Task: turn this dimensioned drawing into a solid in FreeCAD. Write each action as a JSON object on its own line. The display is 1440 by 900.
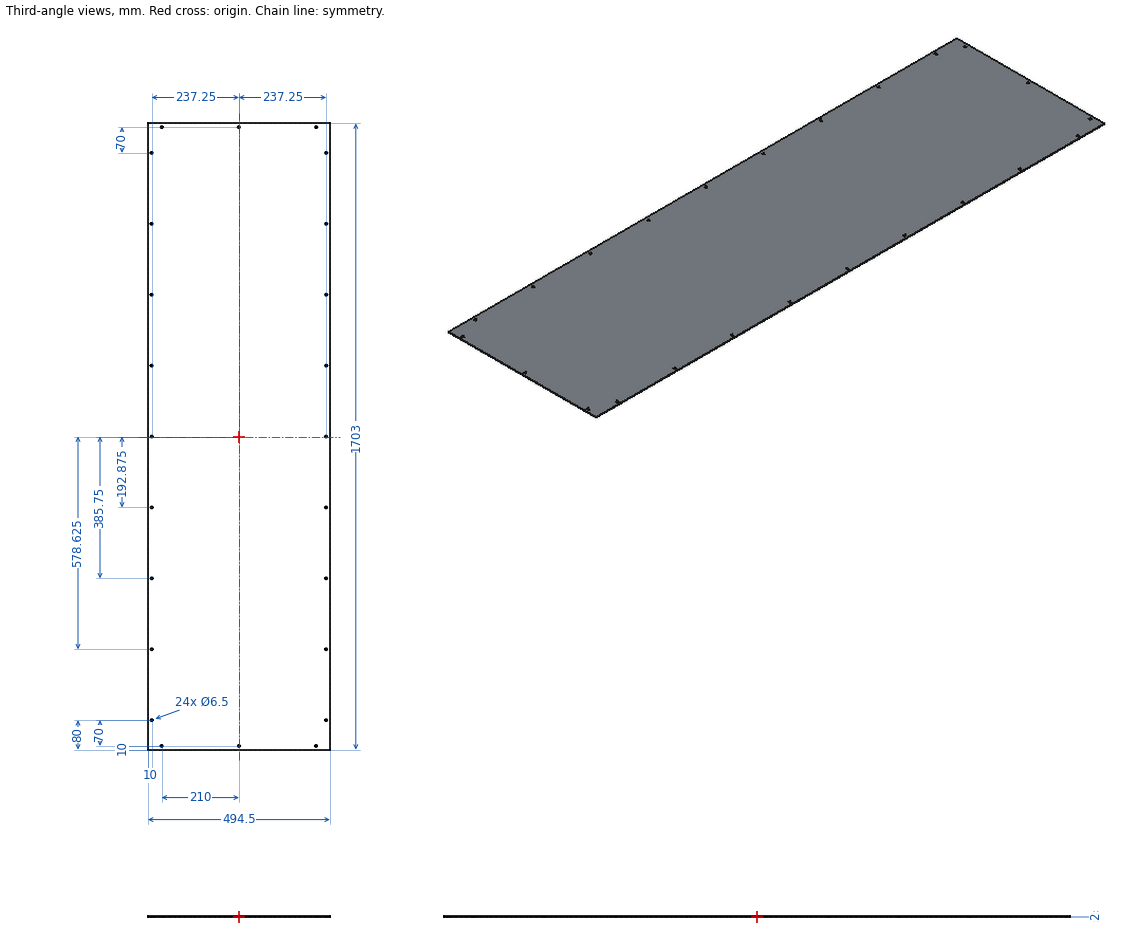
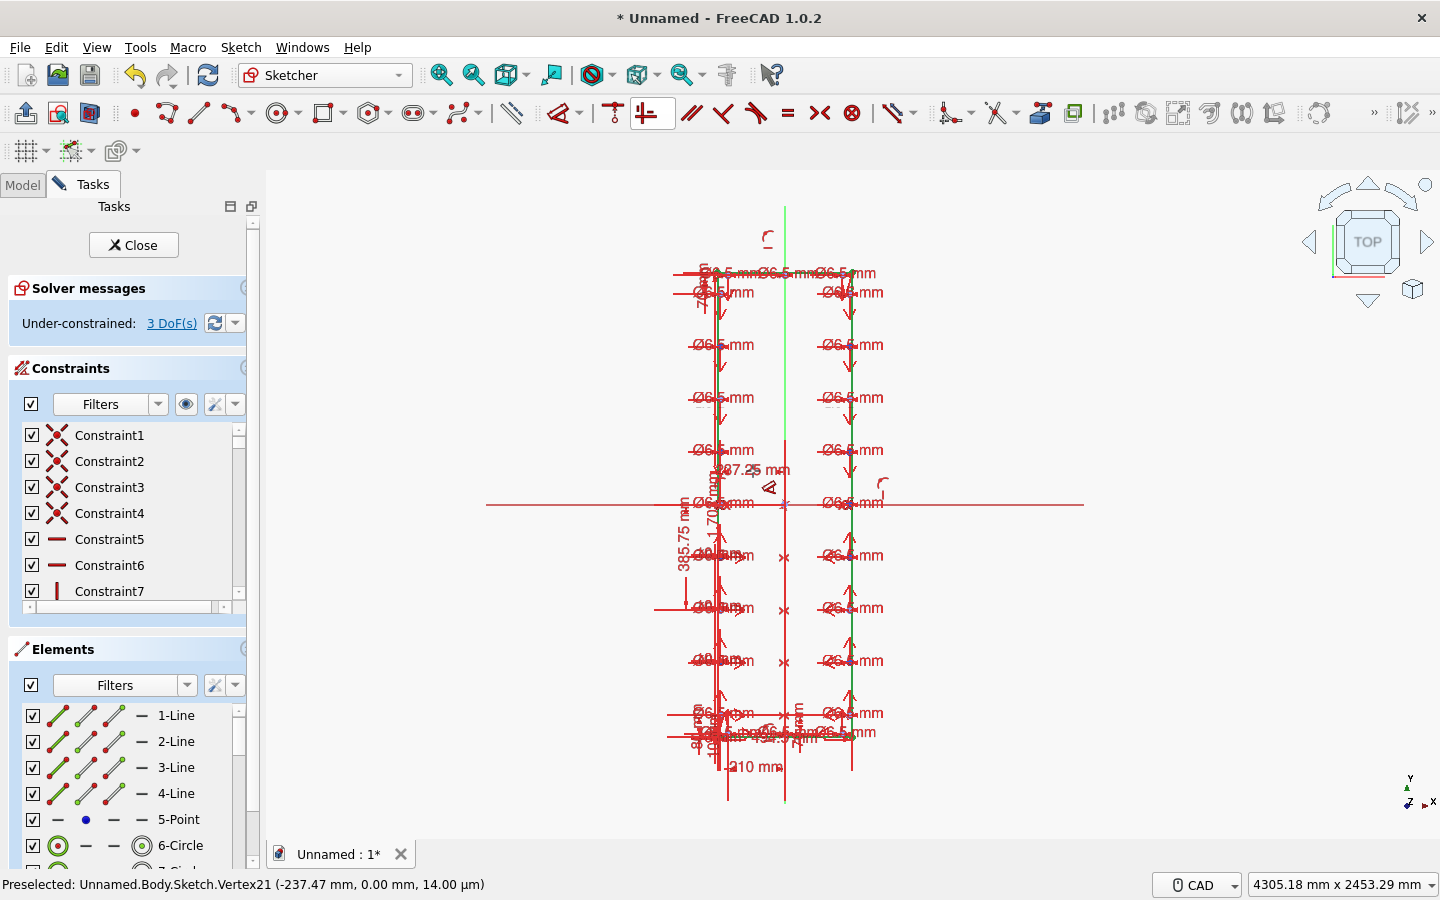
{"action": "left_click", "coordinate": [850, 505]}
{"action": "left_click", "coordinate": [817, 539]}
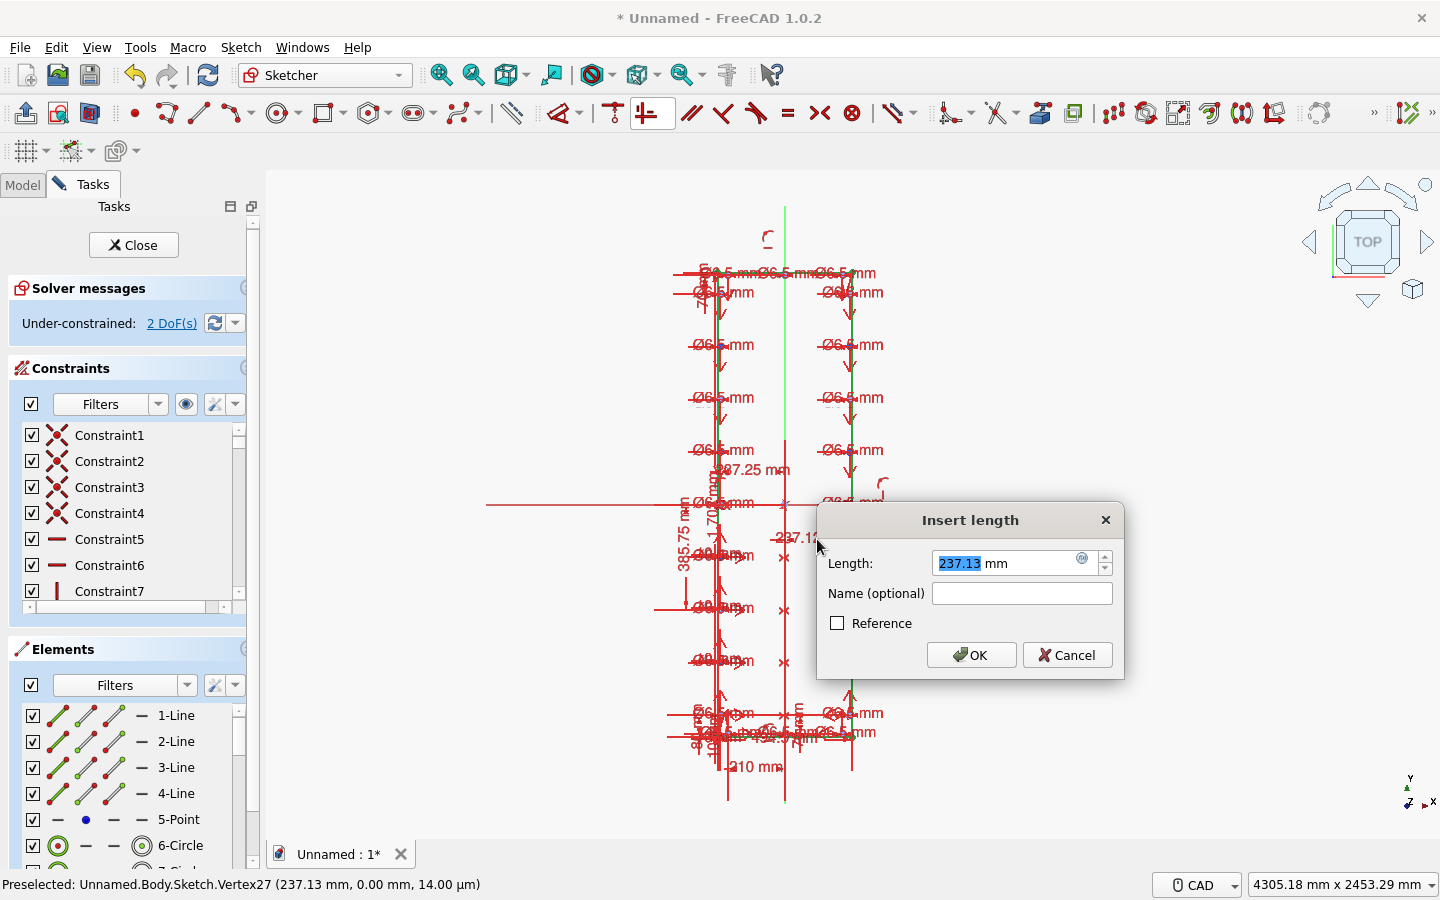
{"action": "type", "text": "237.25"}
{"action": "key", "text": "Return"}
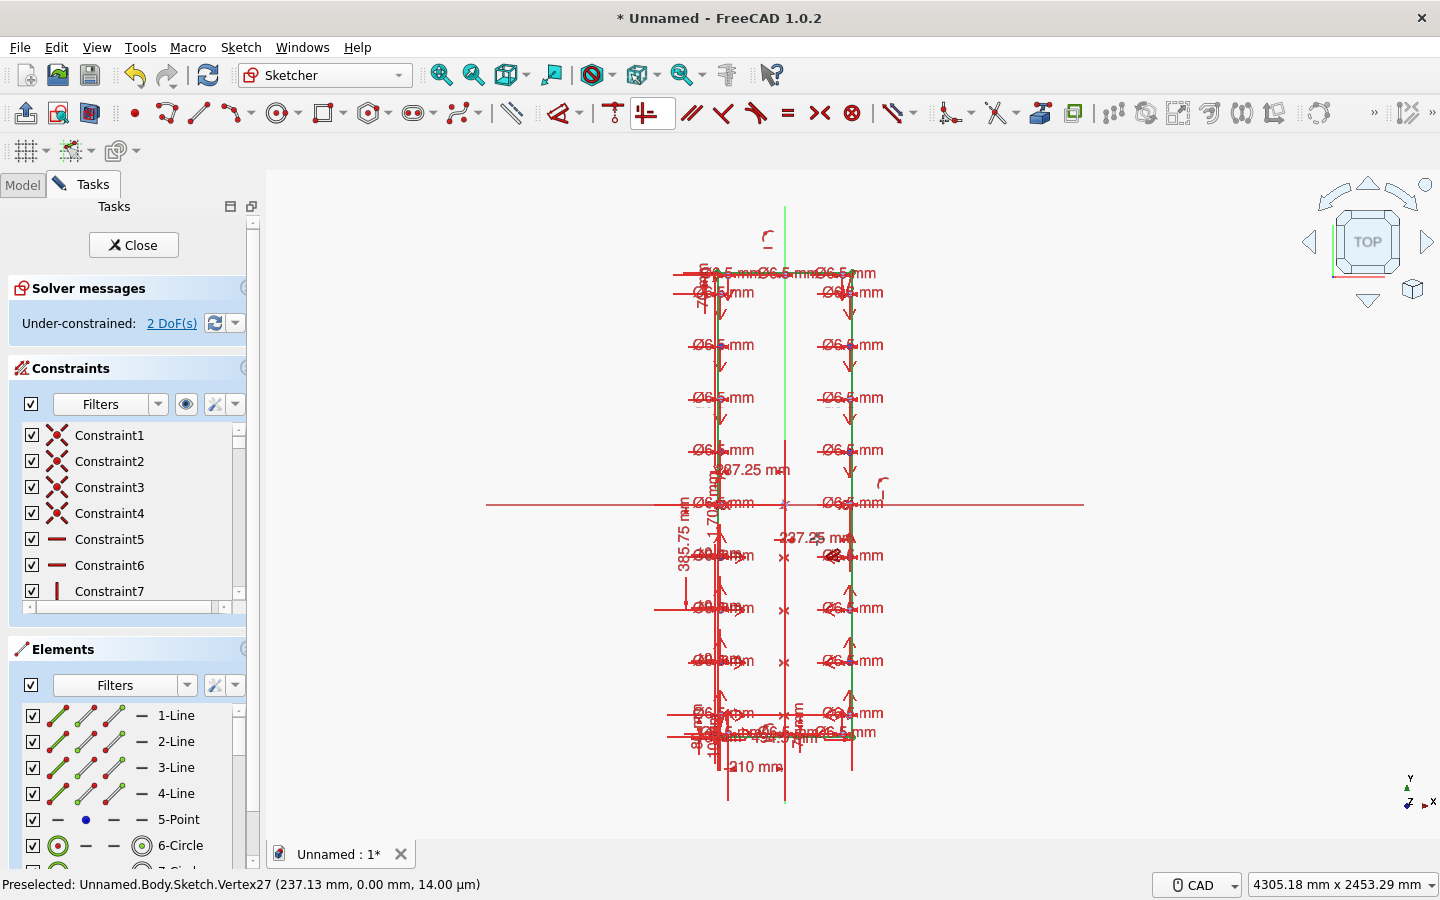
{"action": "left_click", "coordinate": [720, 663]}
{"action": "left_click", "coordinate": [686, 584]}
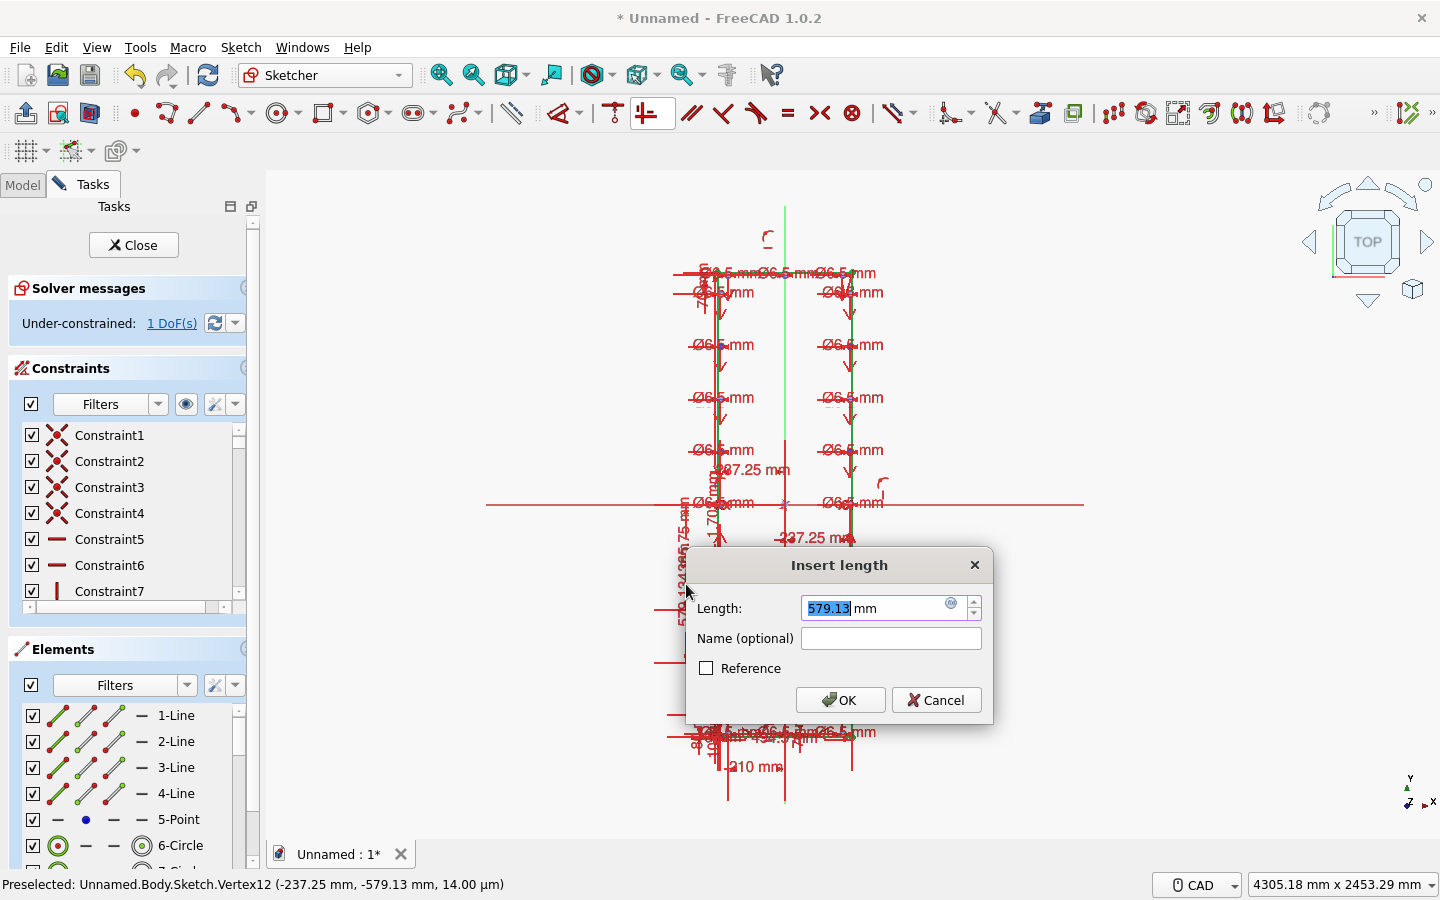
{"action": "type", "text": "578.625"}
{"action": "key", "text": "Return"}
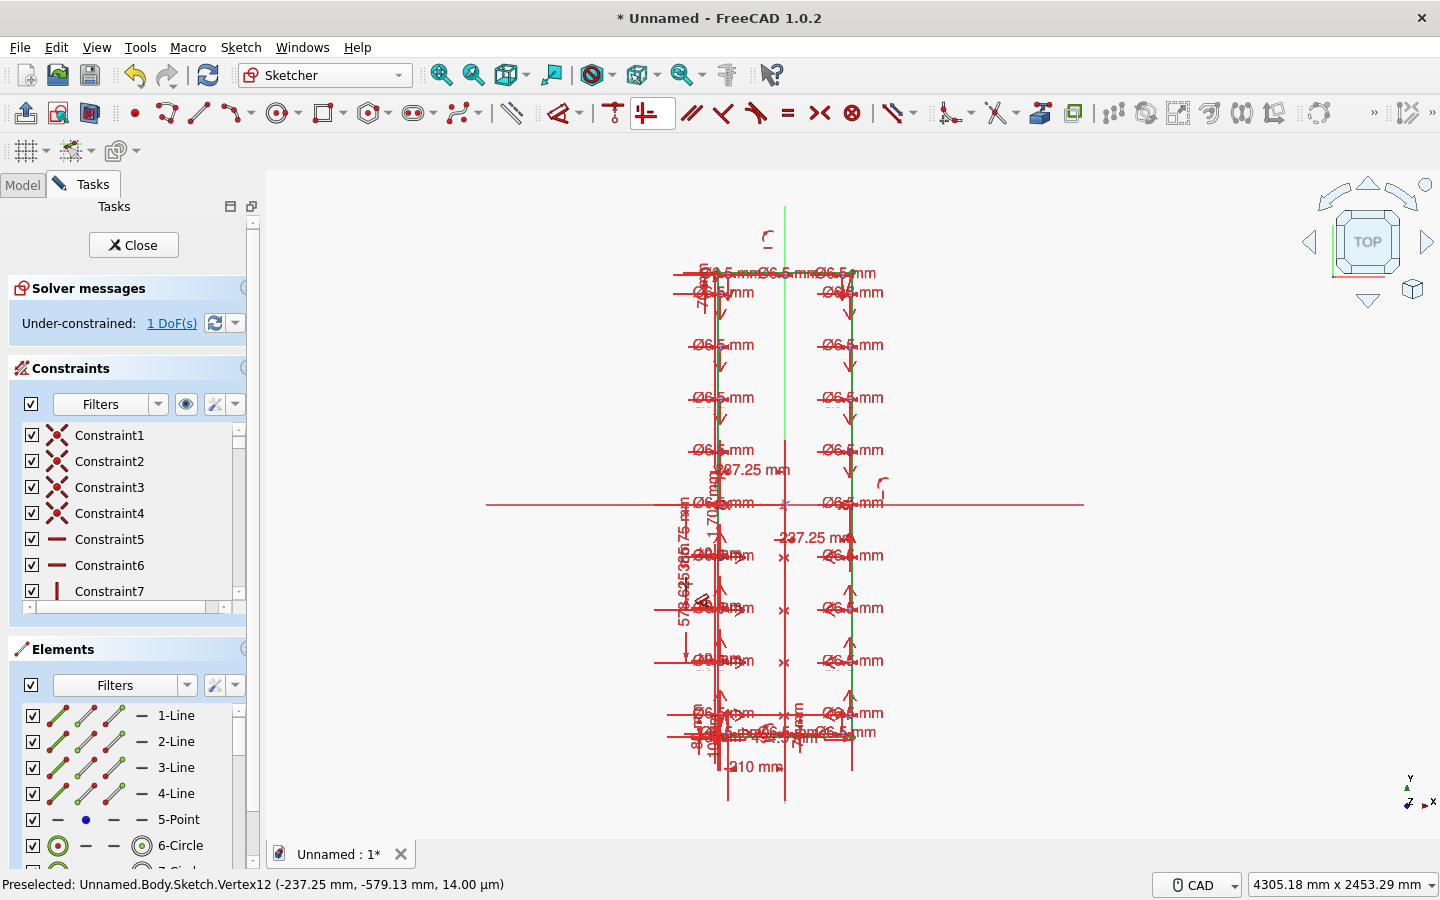
{"action": "left_click", "coordinate": [720, 557]}
{"action": "left_click", "coordinate": [614, 531]}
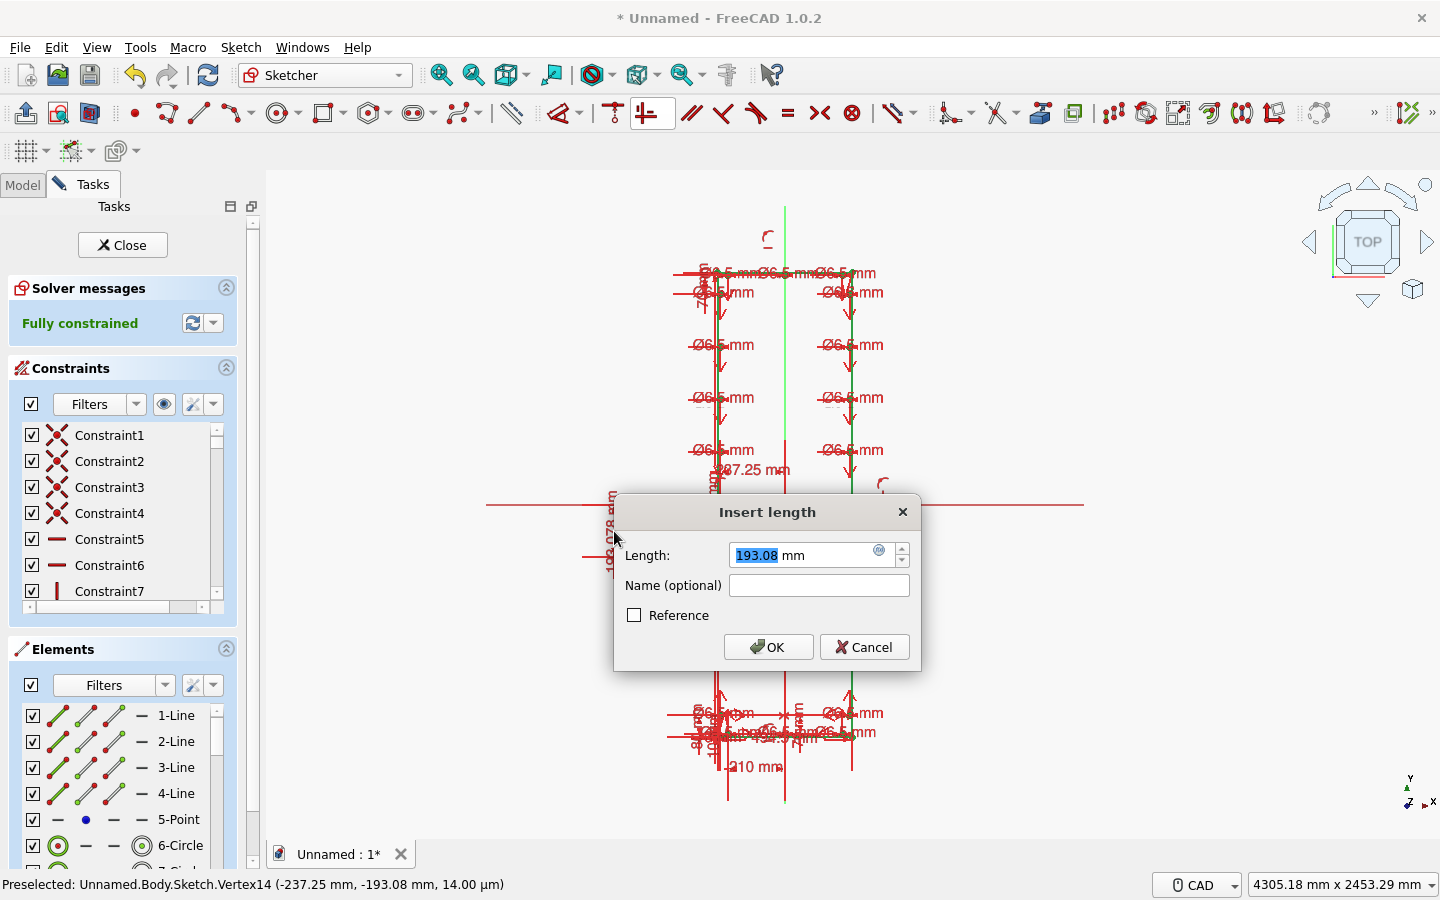
{"action": "type", "text": "192.875"}
{"action": "key", "text": "Return"}
{"action": "key", "text": "Escape"}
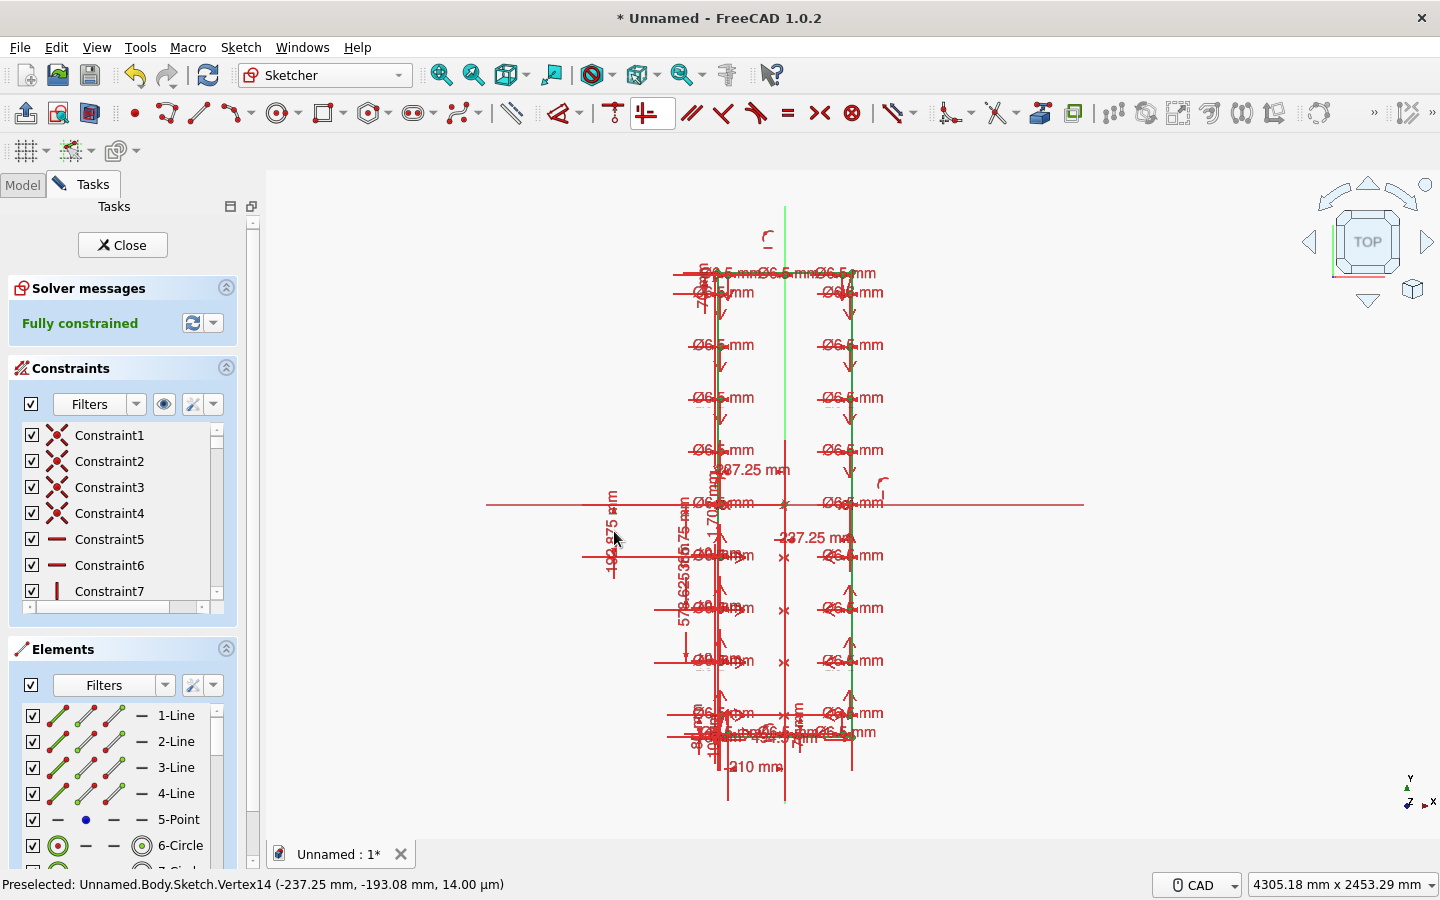
{"action": "left_click", "coordinate": [123, 245]}